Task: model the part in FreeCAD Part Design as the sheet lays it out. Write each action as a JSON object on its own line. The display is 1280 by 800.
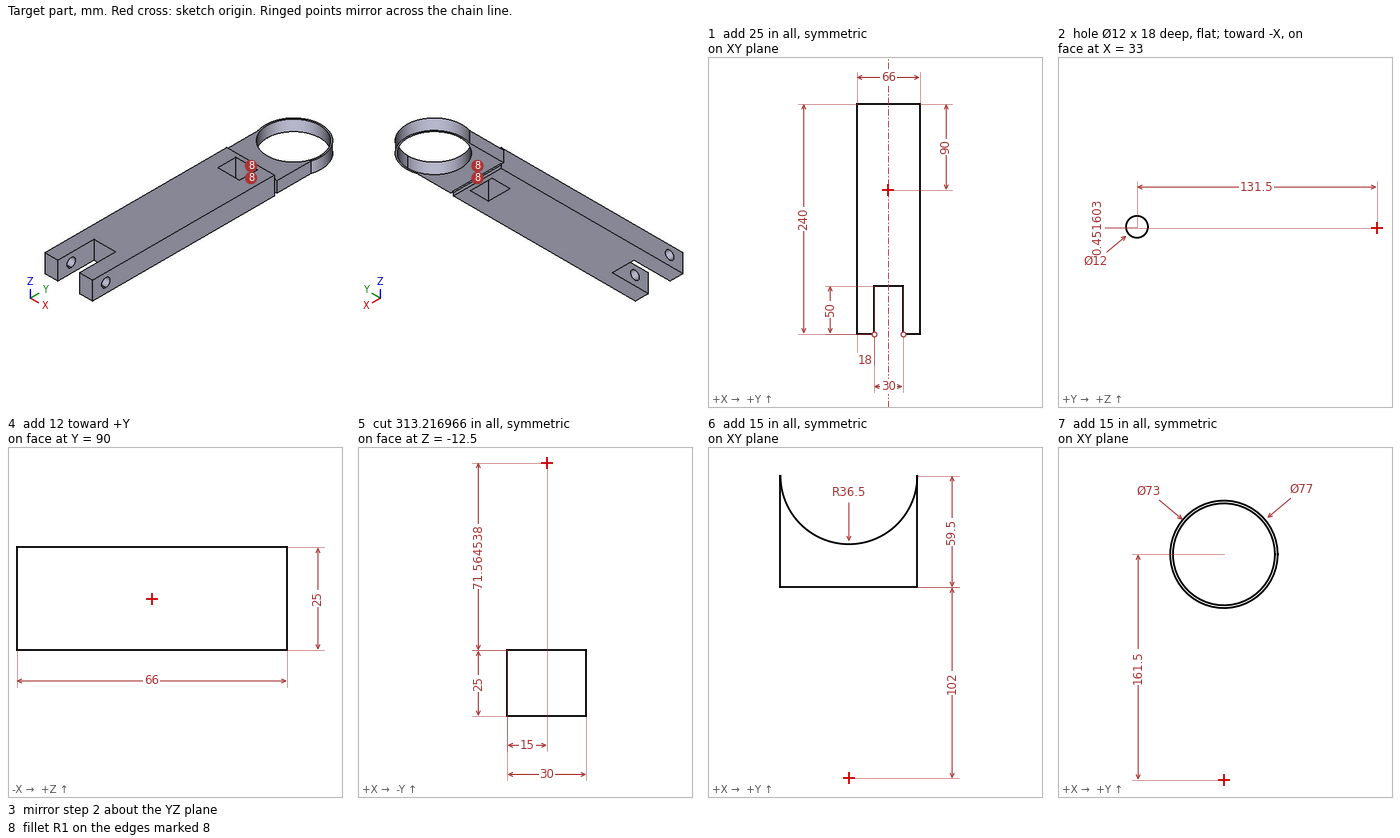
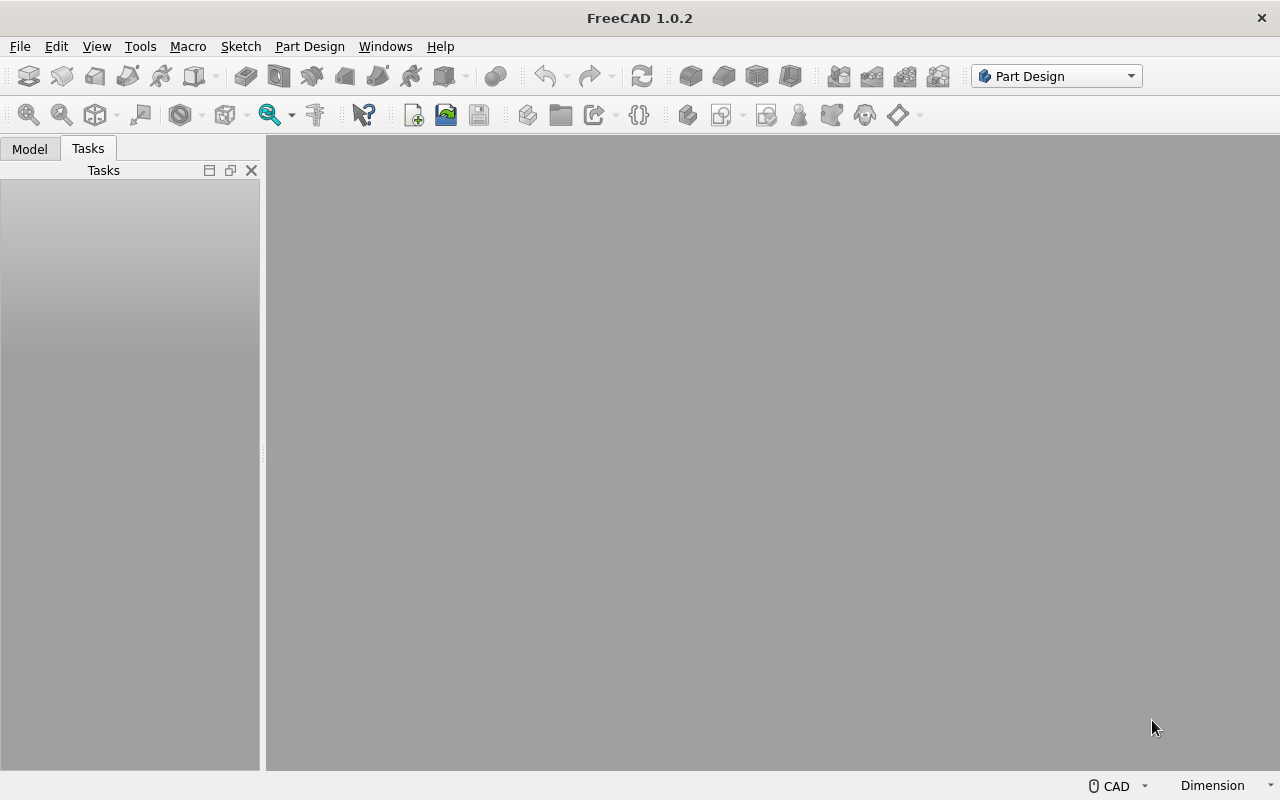
{"action": "left_click", "coordinate": [413, 116]}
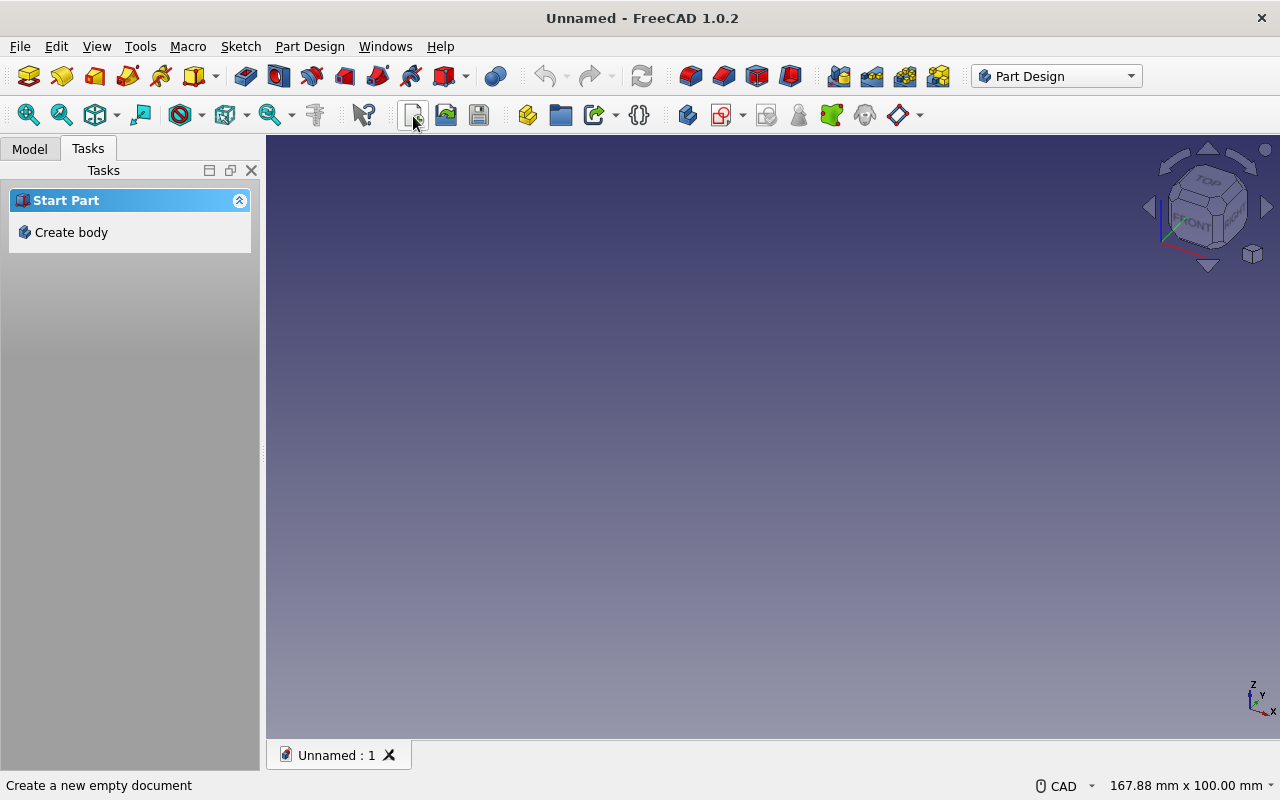
{"action": "left_click", "coordinate": [720, 116]}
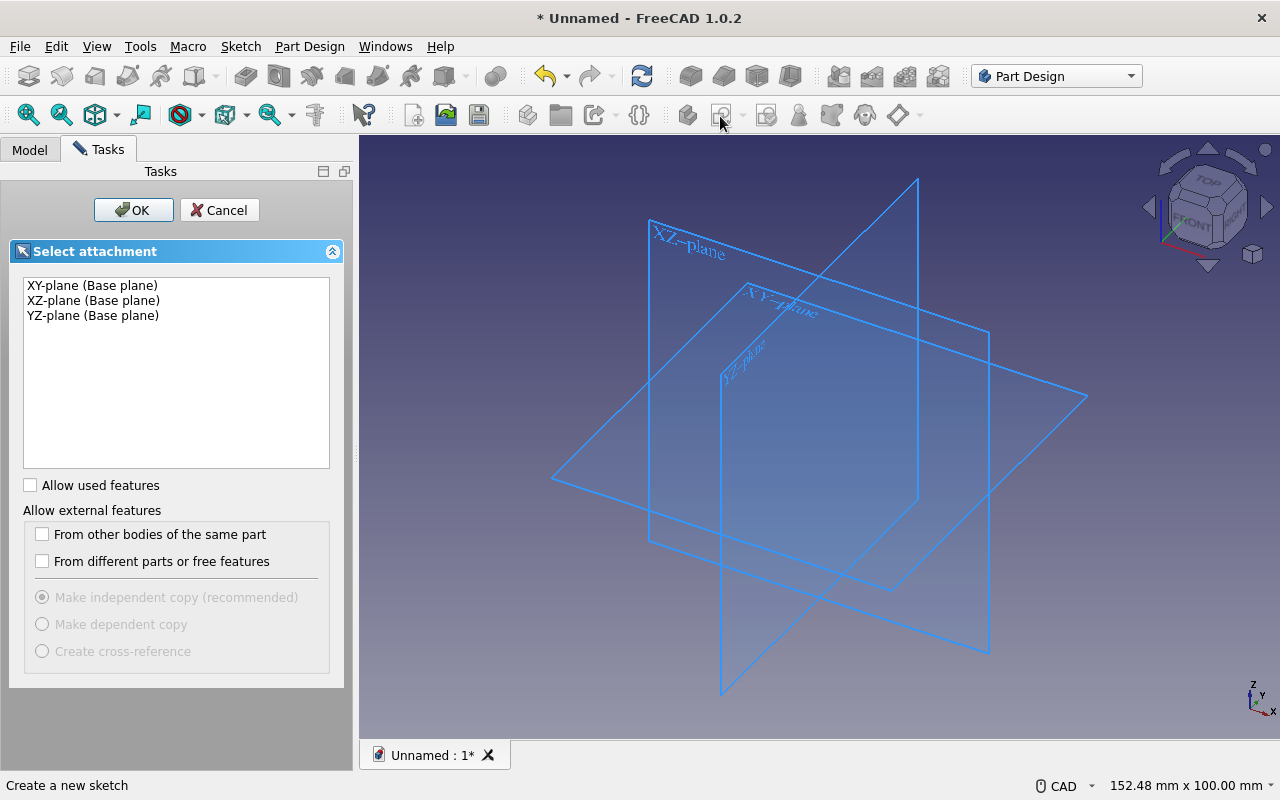
{"action": "left_click", "coordinate": [84, 286]}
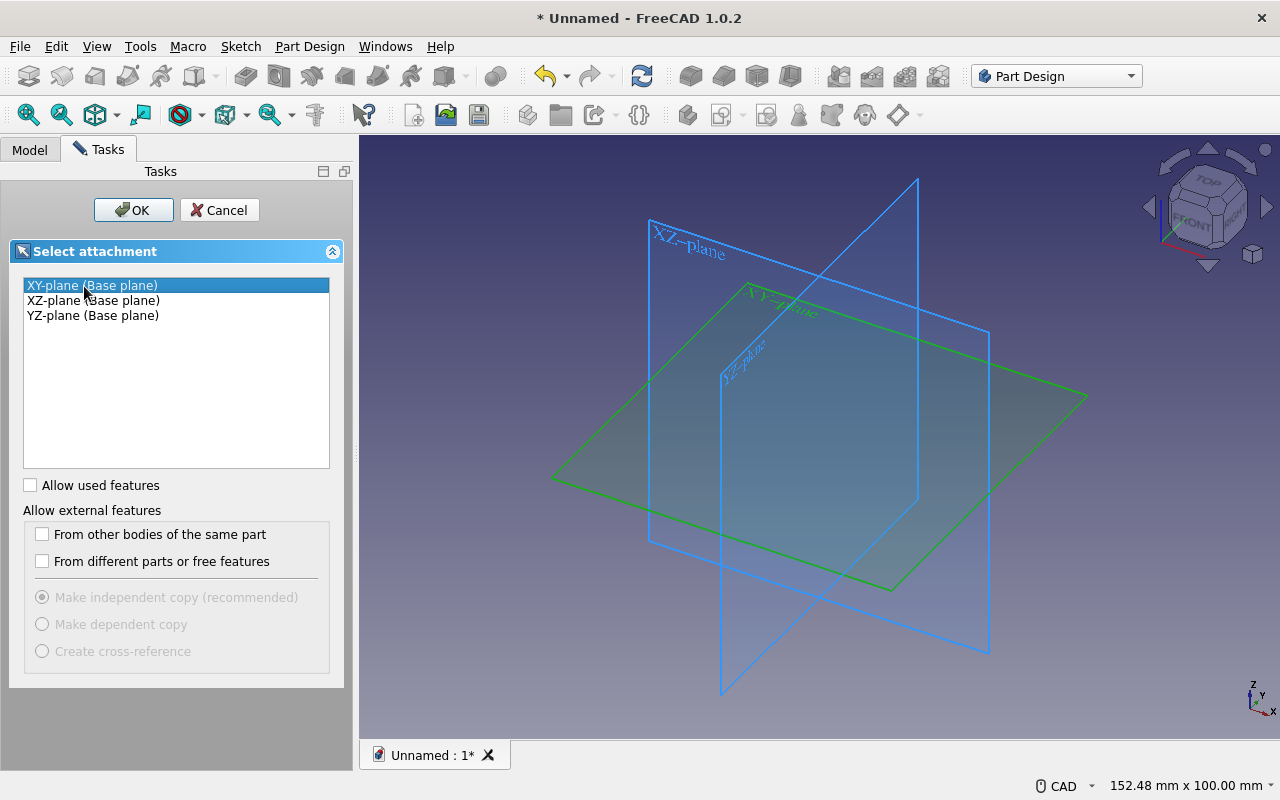
{"action": "left_click", "coordinate": [134, 210]}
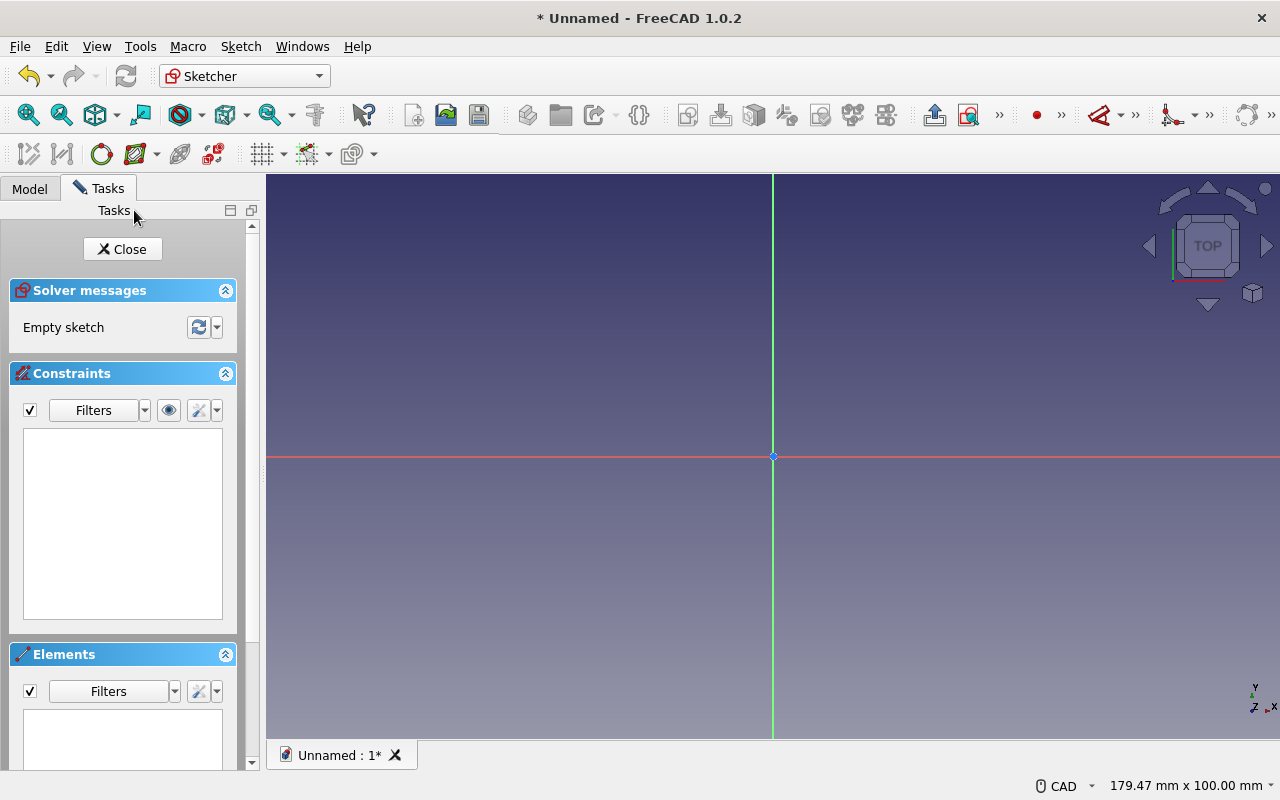
{"action": "scroll", "coordinate": [682, 401], "scroll_direction": "down", "scroll_amount": 7}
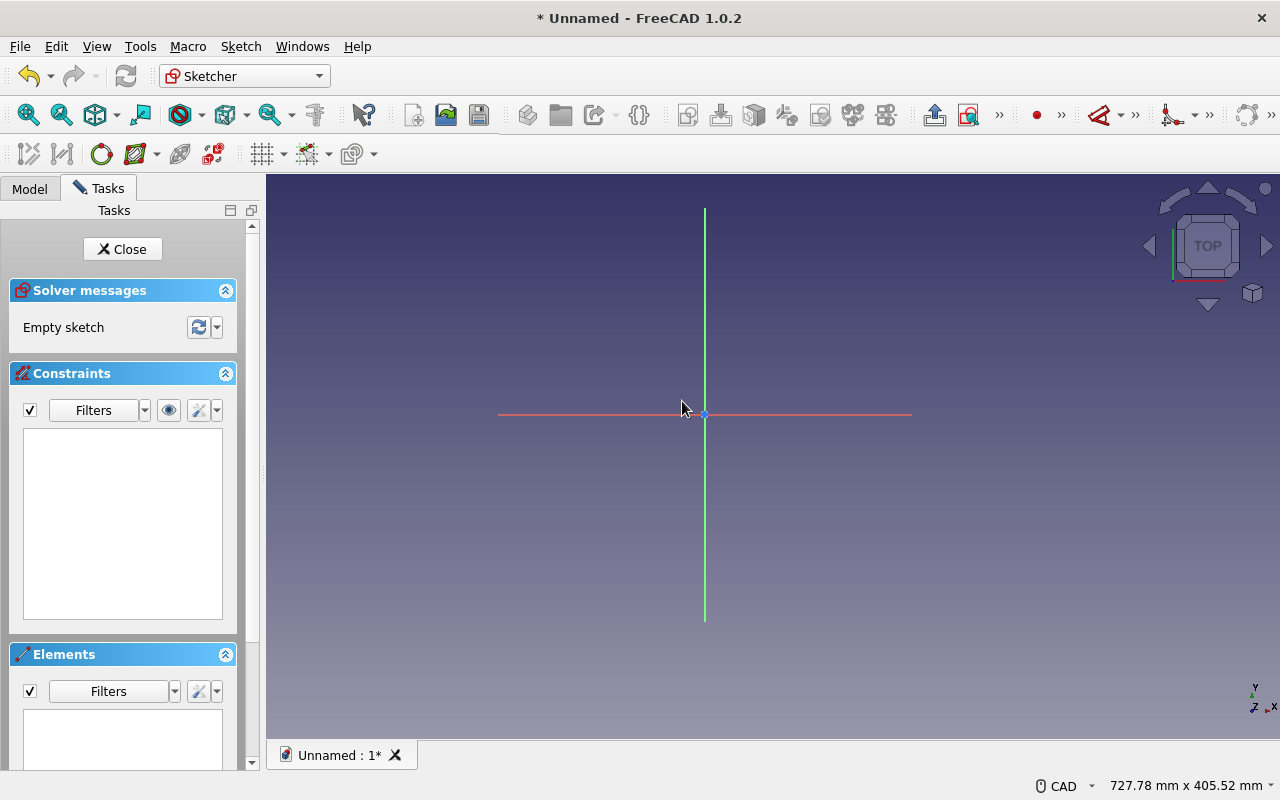
{"action": "key", "text": "g m"}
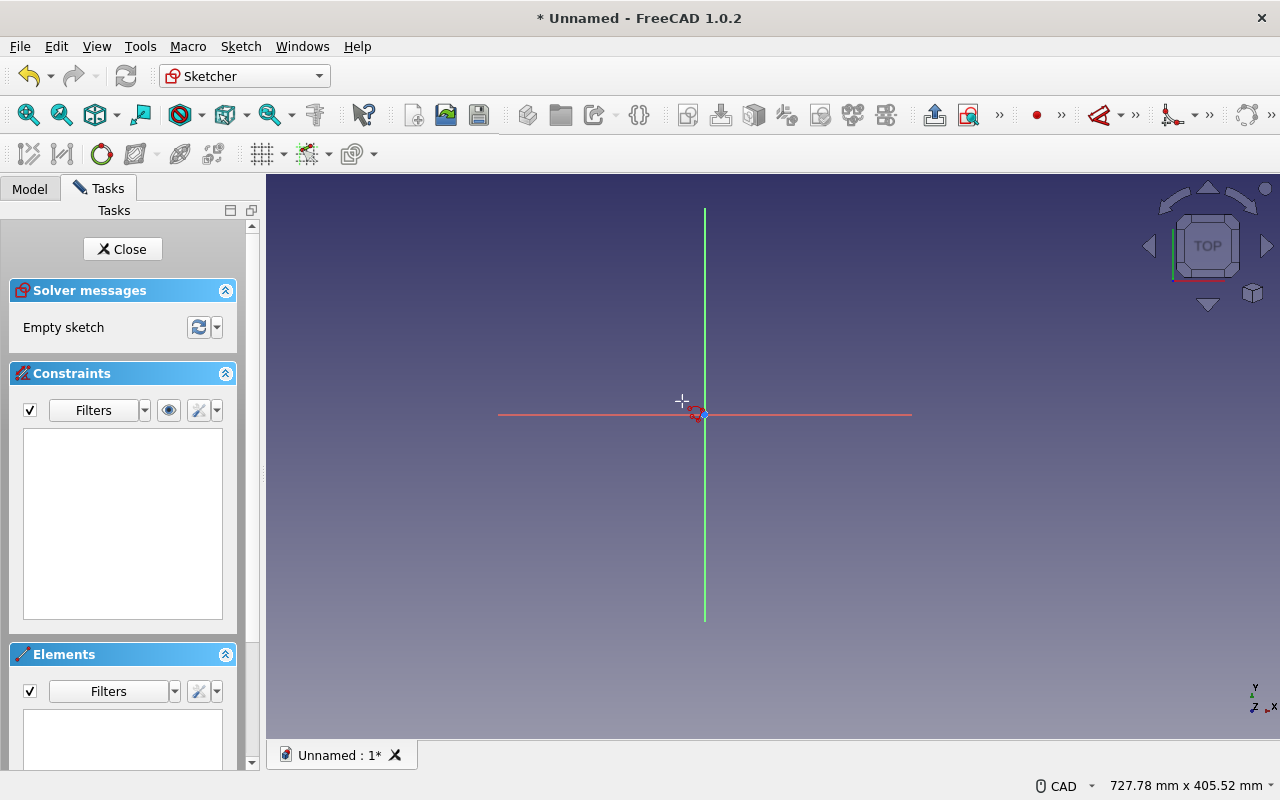
{"action": "left_click", "coordinate": [751, 290]}
{"action": "left_click", "coordinate": [659, 290]}
{"action": "left_click", "coordinate": [659, 624]}
{"action": "left_click", "coordinate": [684, 624]}
{"action": "left_click", "coordinate": [684, 554]}
{"action": "left_click", "coordinate": [726, 554]}
{"action": "left_click", "coordinate": [726, 624]}
{"action": "left_click", "coordinate": [751, 624]}
{"action": "left_click", "coordinate": [751, 291]}
{"action": "key", "text": "Escape"}
{"action": "key", "text": "Escape"}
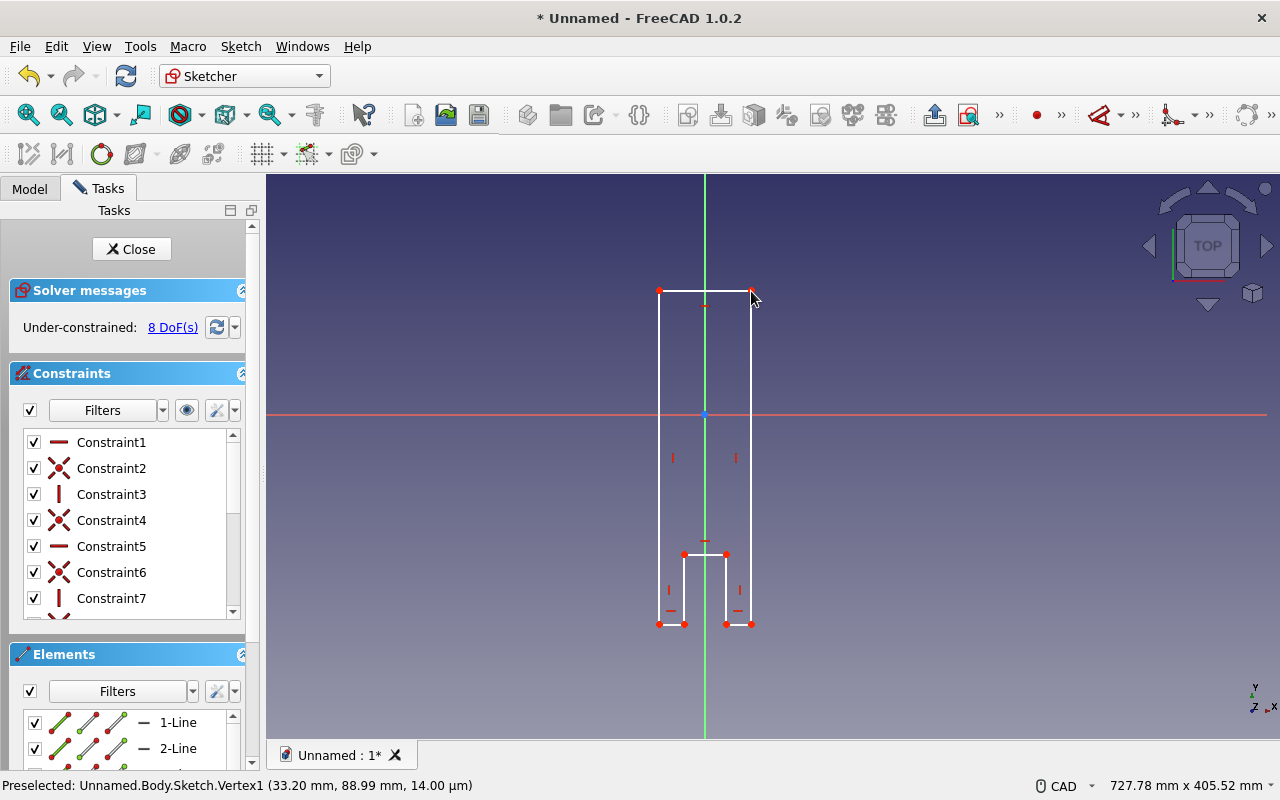
{"action": "left_click", "coordinate": [684, 625]}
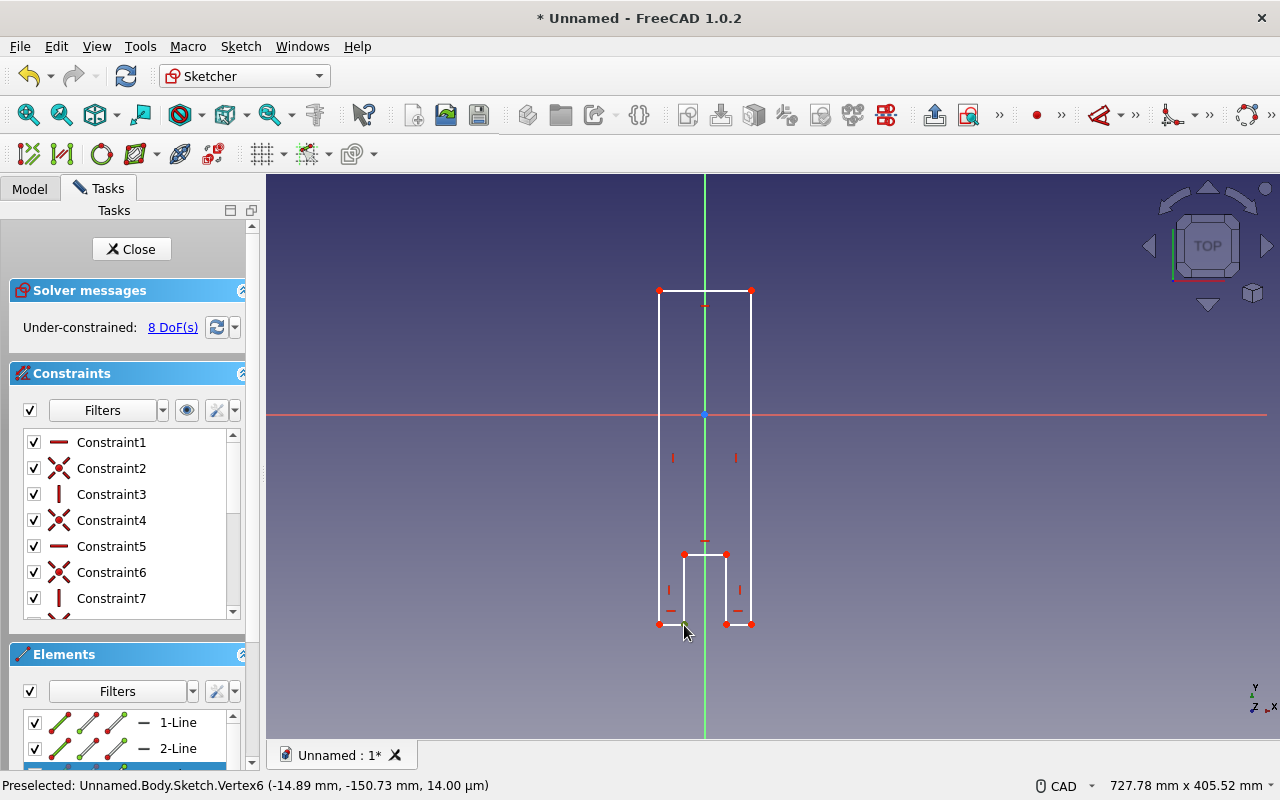
{"action": "left_click", "coordinate": [726, 625]}